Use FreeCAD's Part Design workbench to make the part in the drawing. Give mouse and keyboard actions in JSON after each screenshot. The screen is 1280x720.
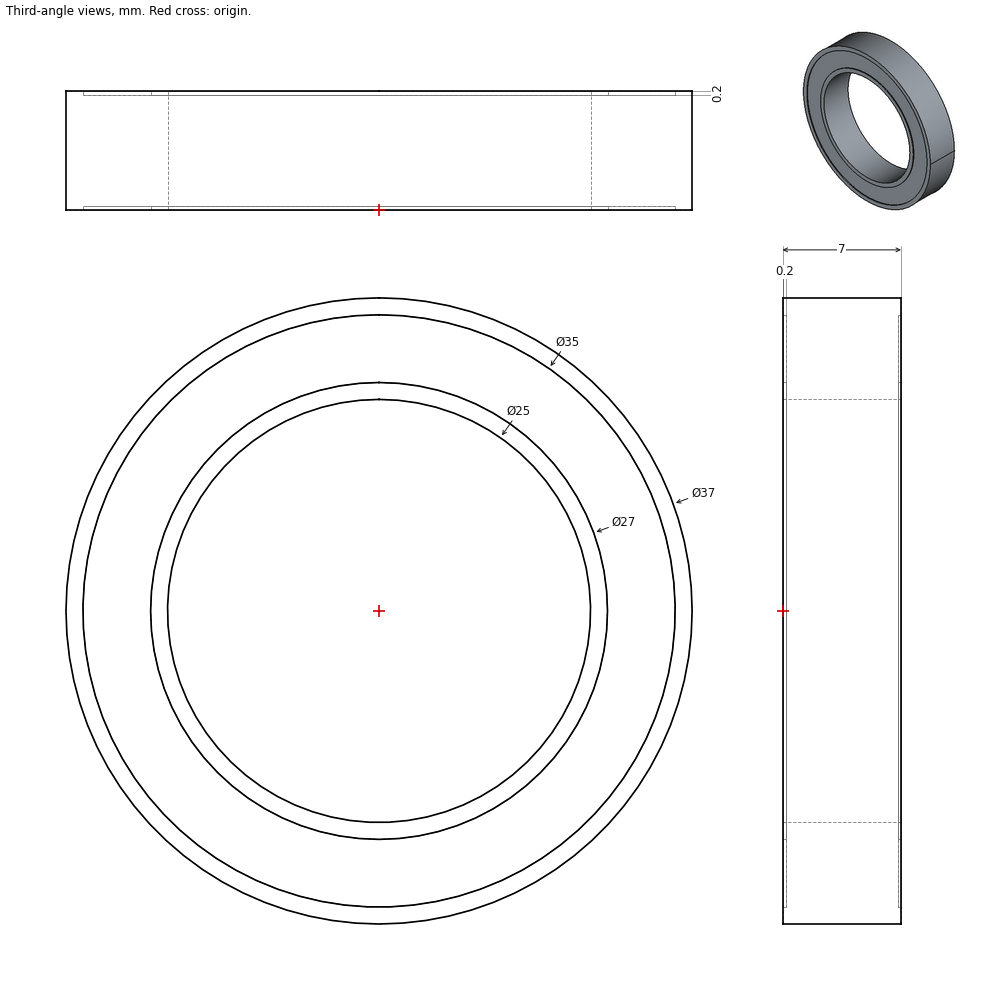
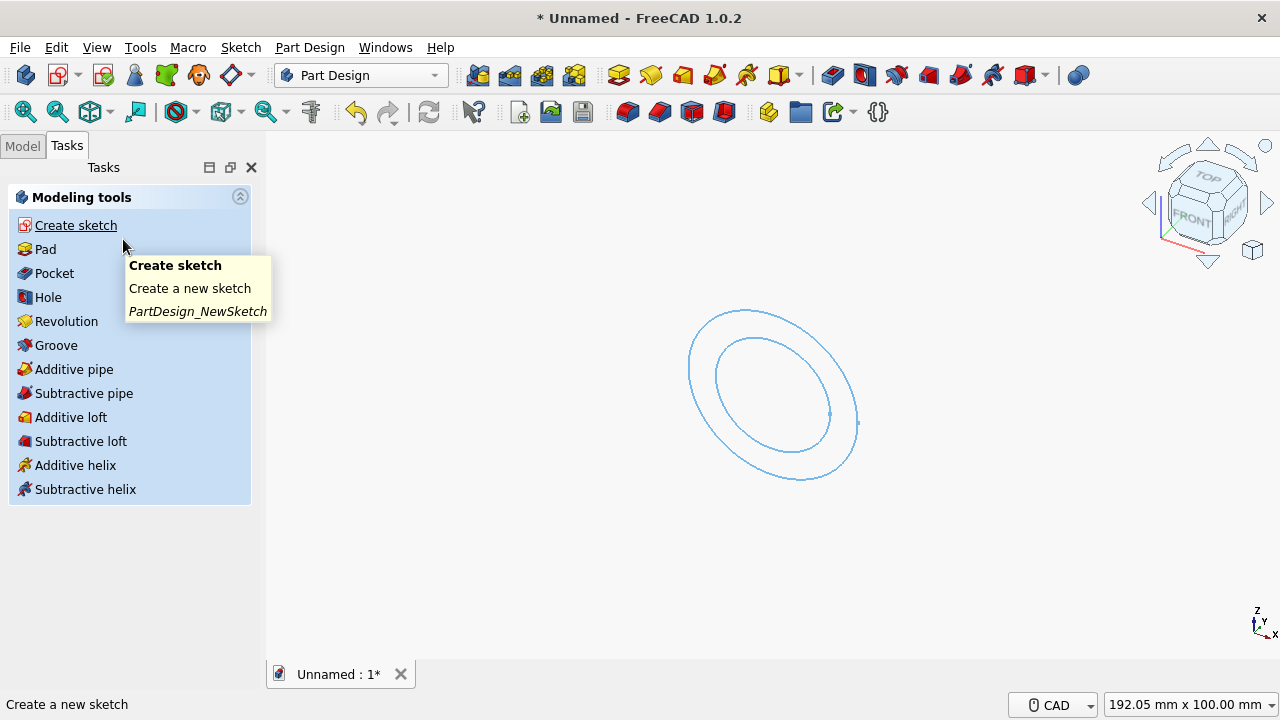
{"action": "left_click", "coordinate": [620, 76]}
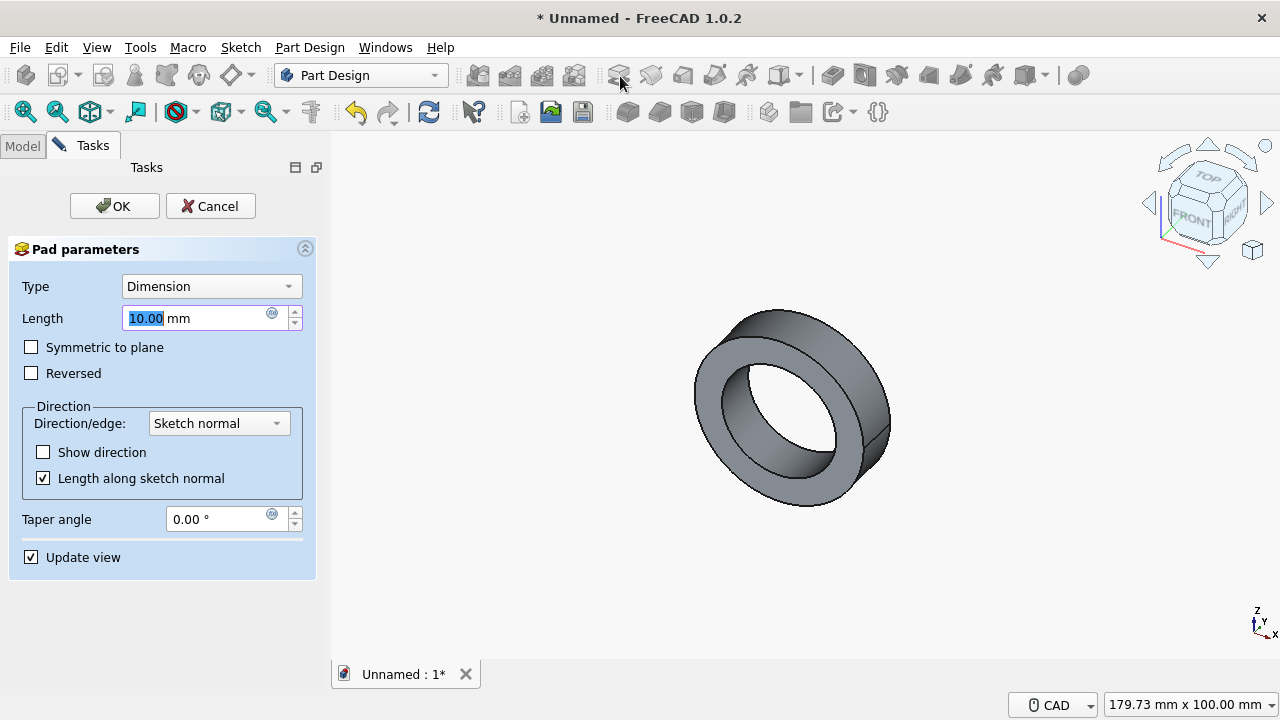
{"action": "type", "text": "7"}
{"action": "key", "text": "Tab"}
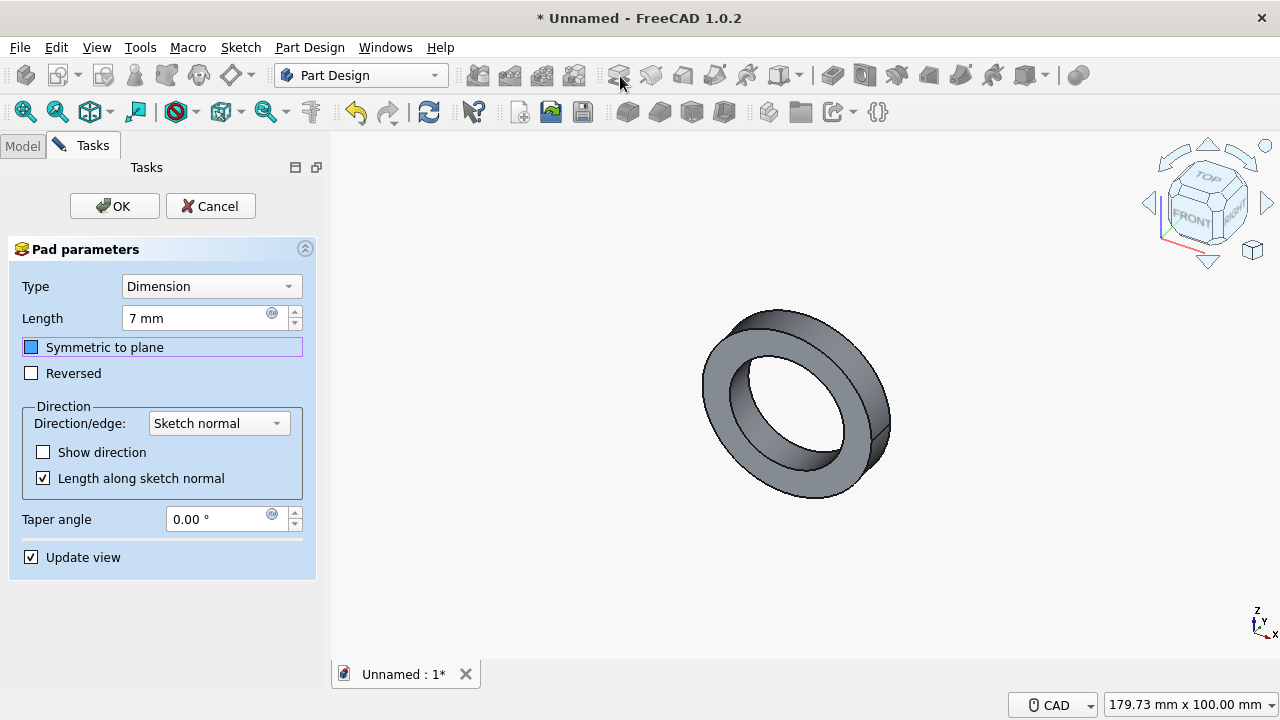
{"action": "left_click", "coordinate": [30, 373]}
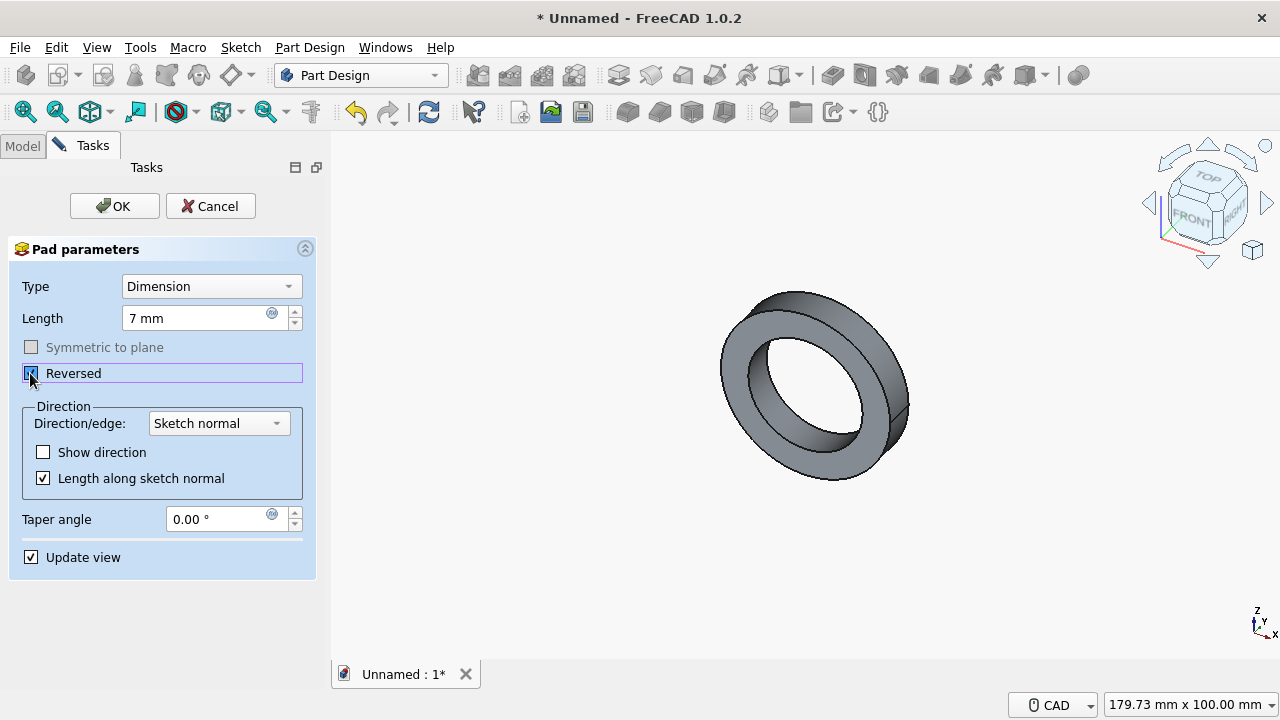
{"action": "left_click", "coordinate": [115, 206]}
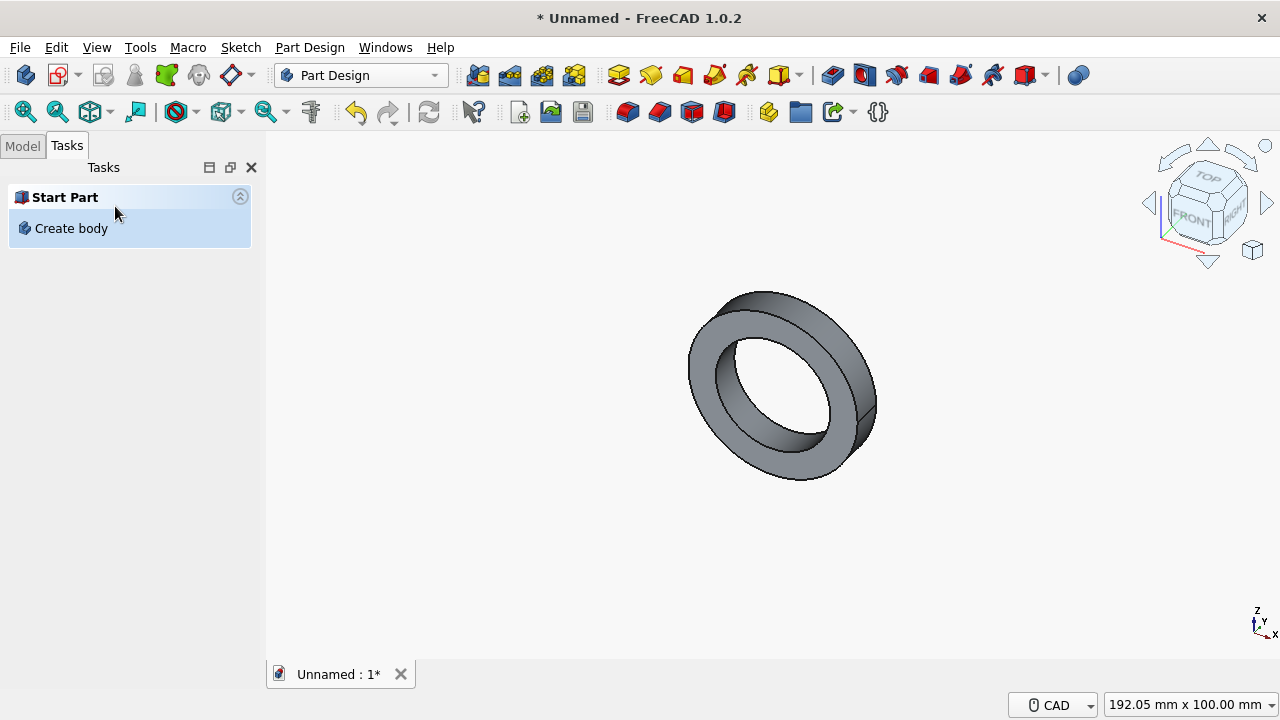
{"action": "key", "text": "v f"}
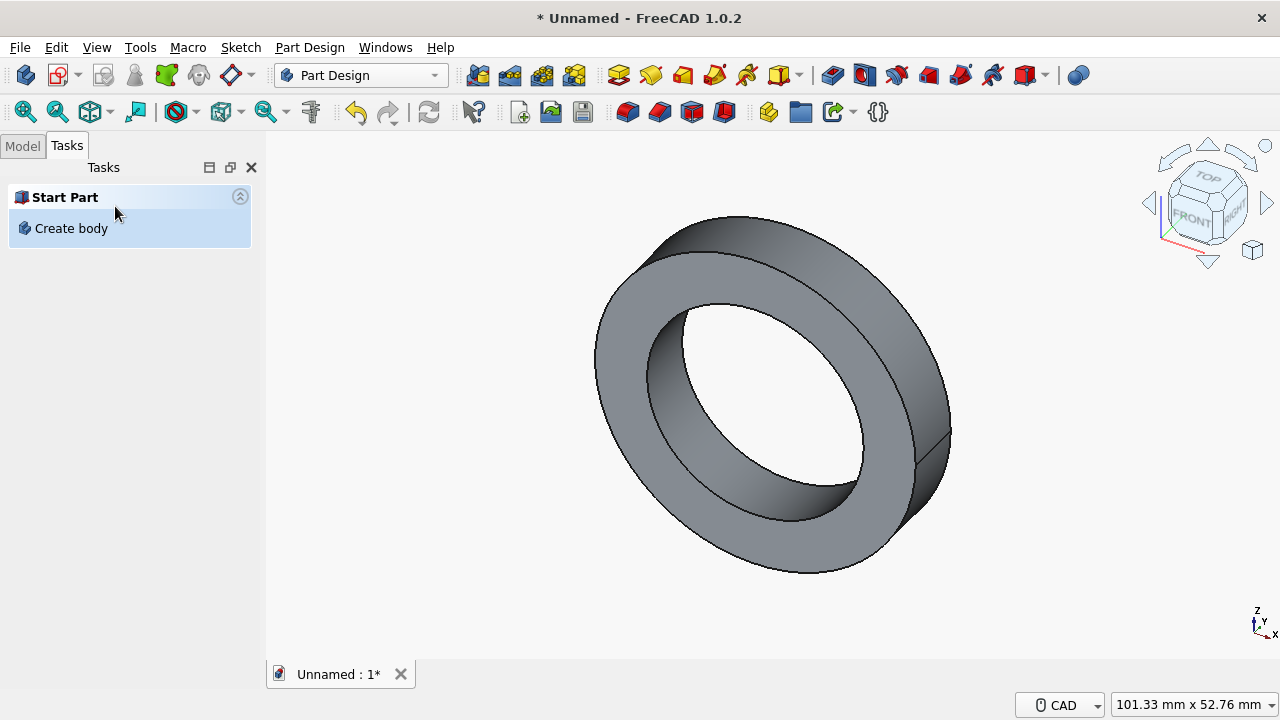
{"action": "key", "text": "4"}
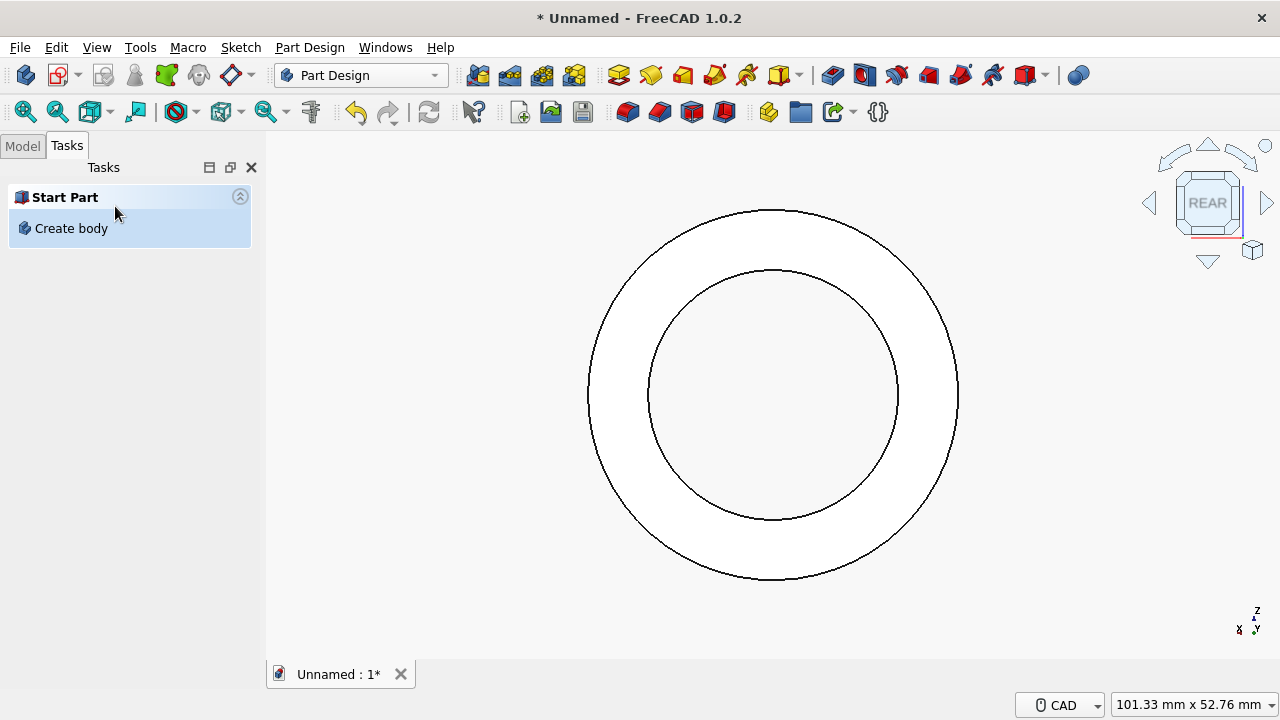
{"action": "left_click", "coordinate": [614, 394]}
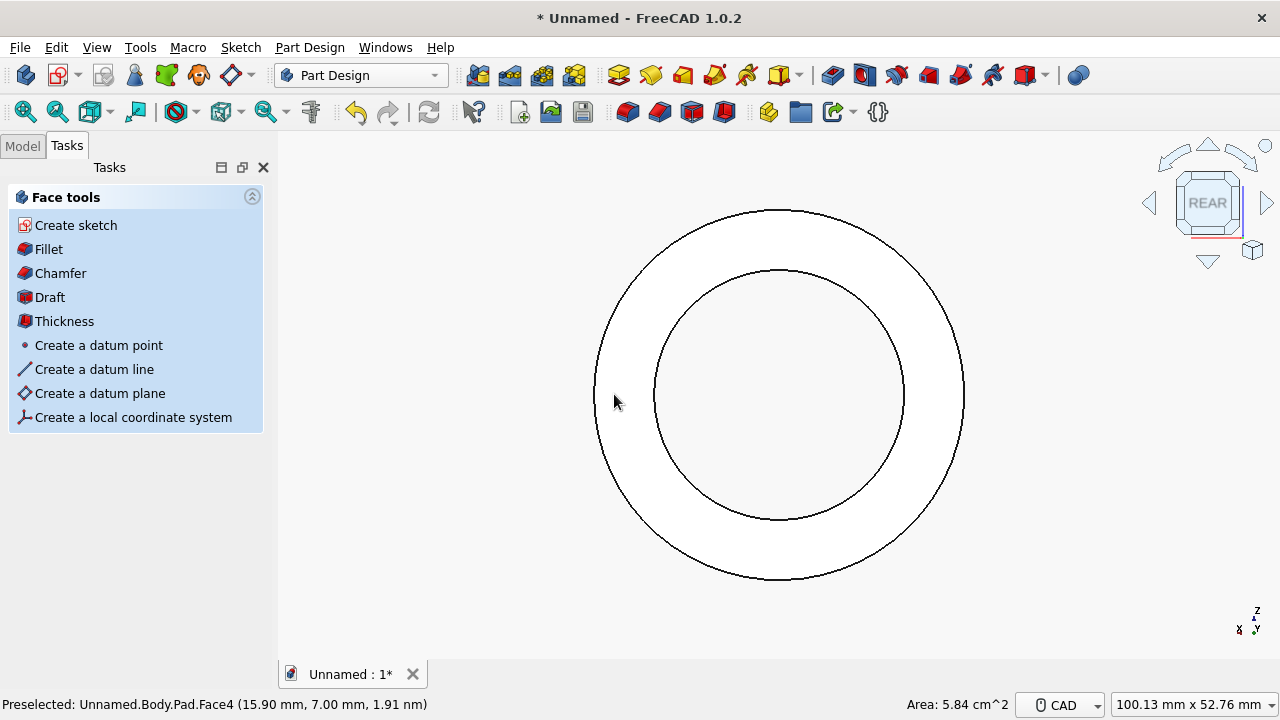
{"action": "left_click", "coordinate": [58, 76]}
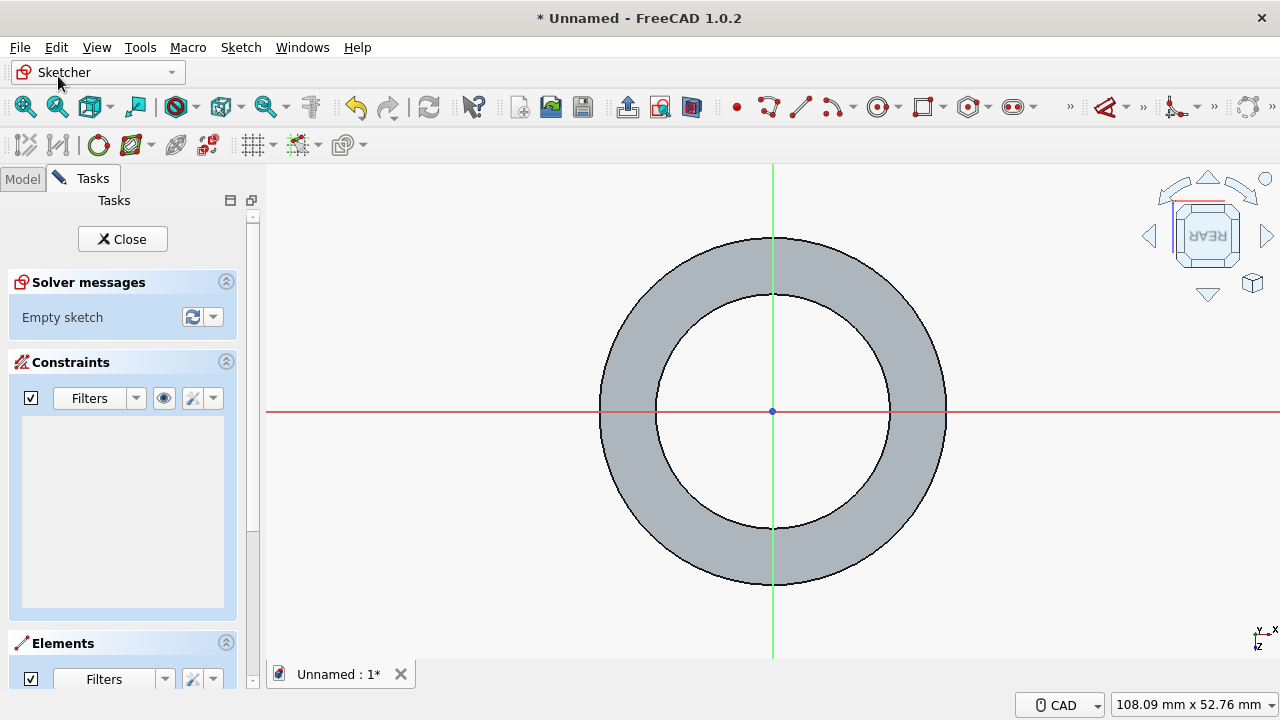
{"action": "key", "text": "g c"}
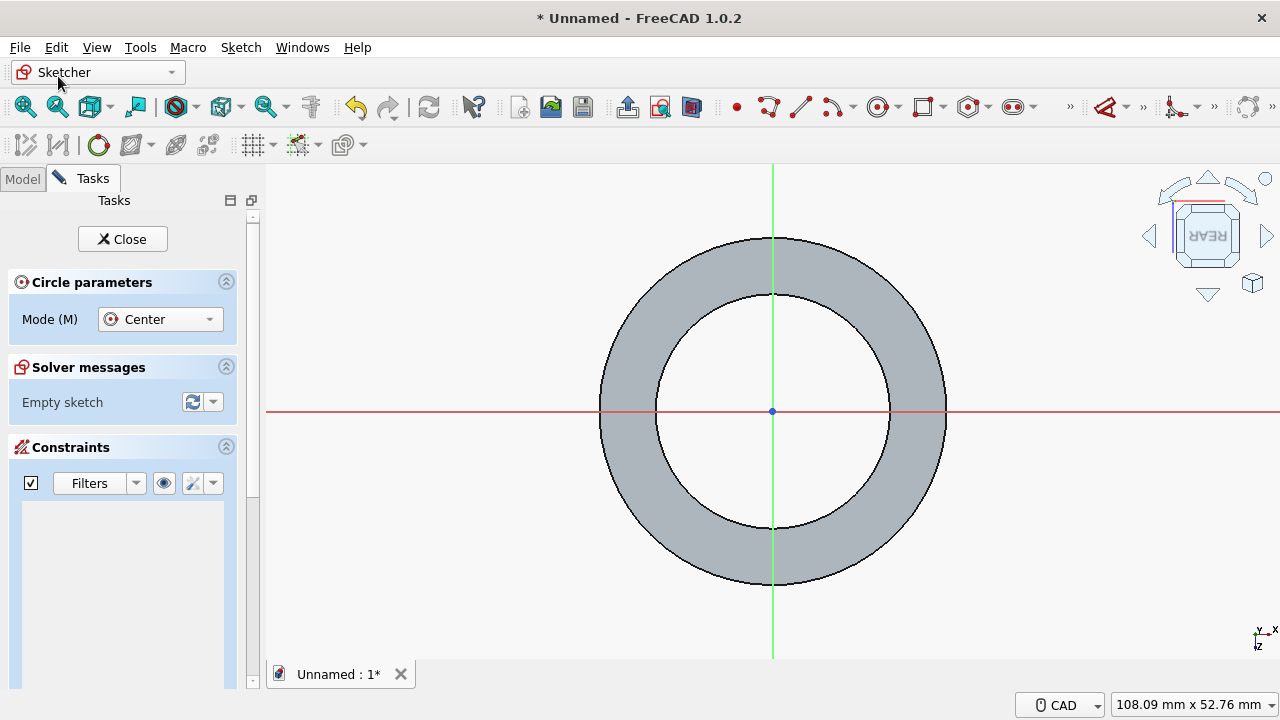
{"action": "left_click", "coordinate": [773, 411]}
{"action": "mouse_move", "coordinate": [889, 295]}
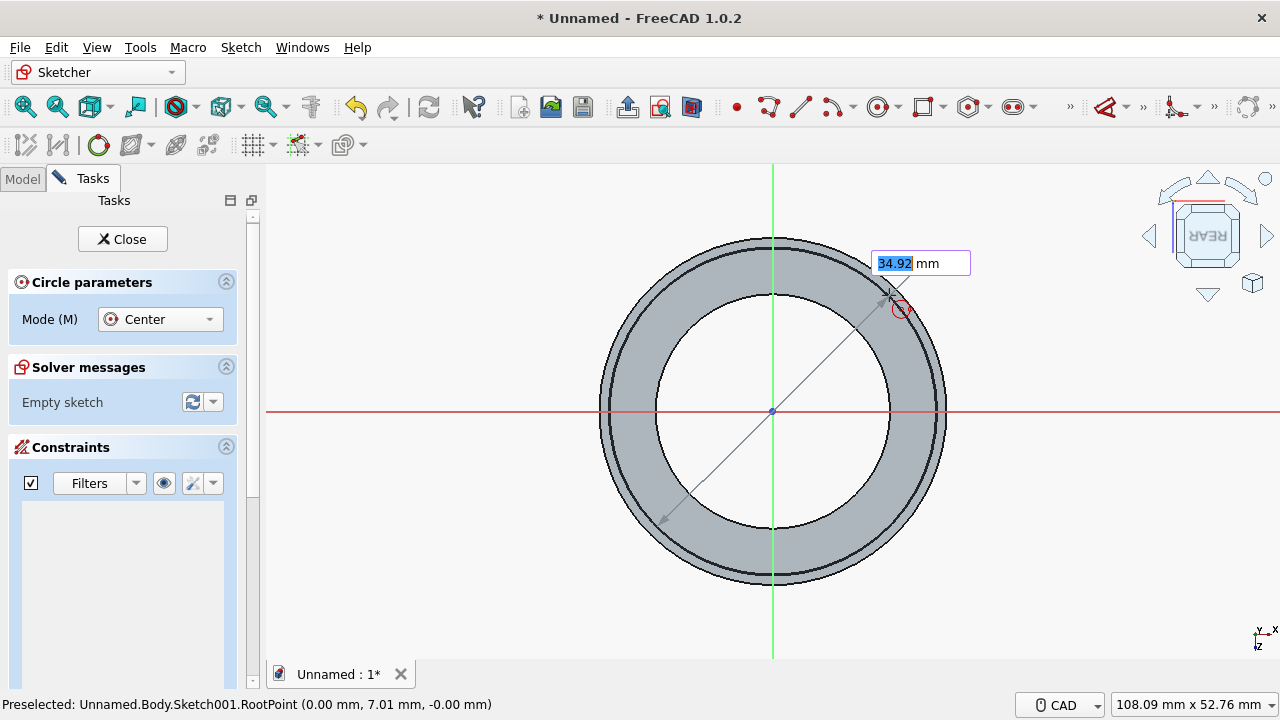
{"action": "type", "text": "35"}
{"action": "key", "text": "Return"}